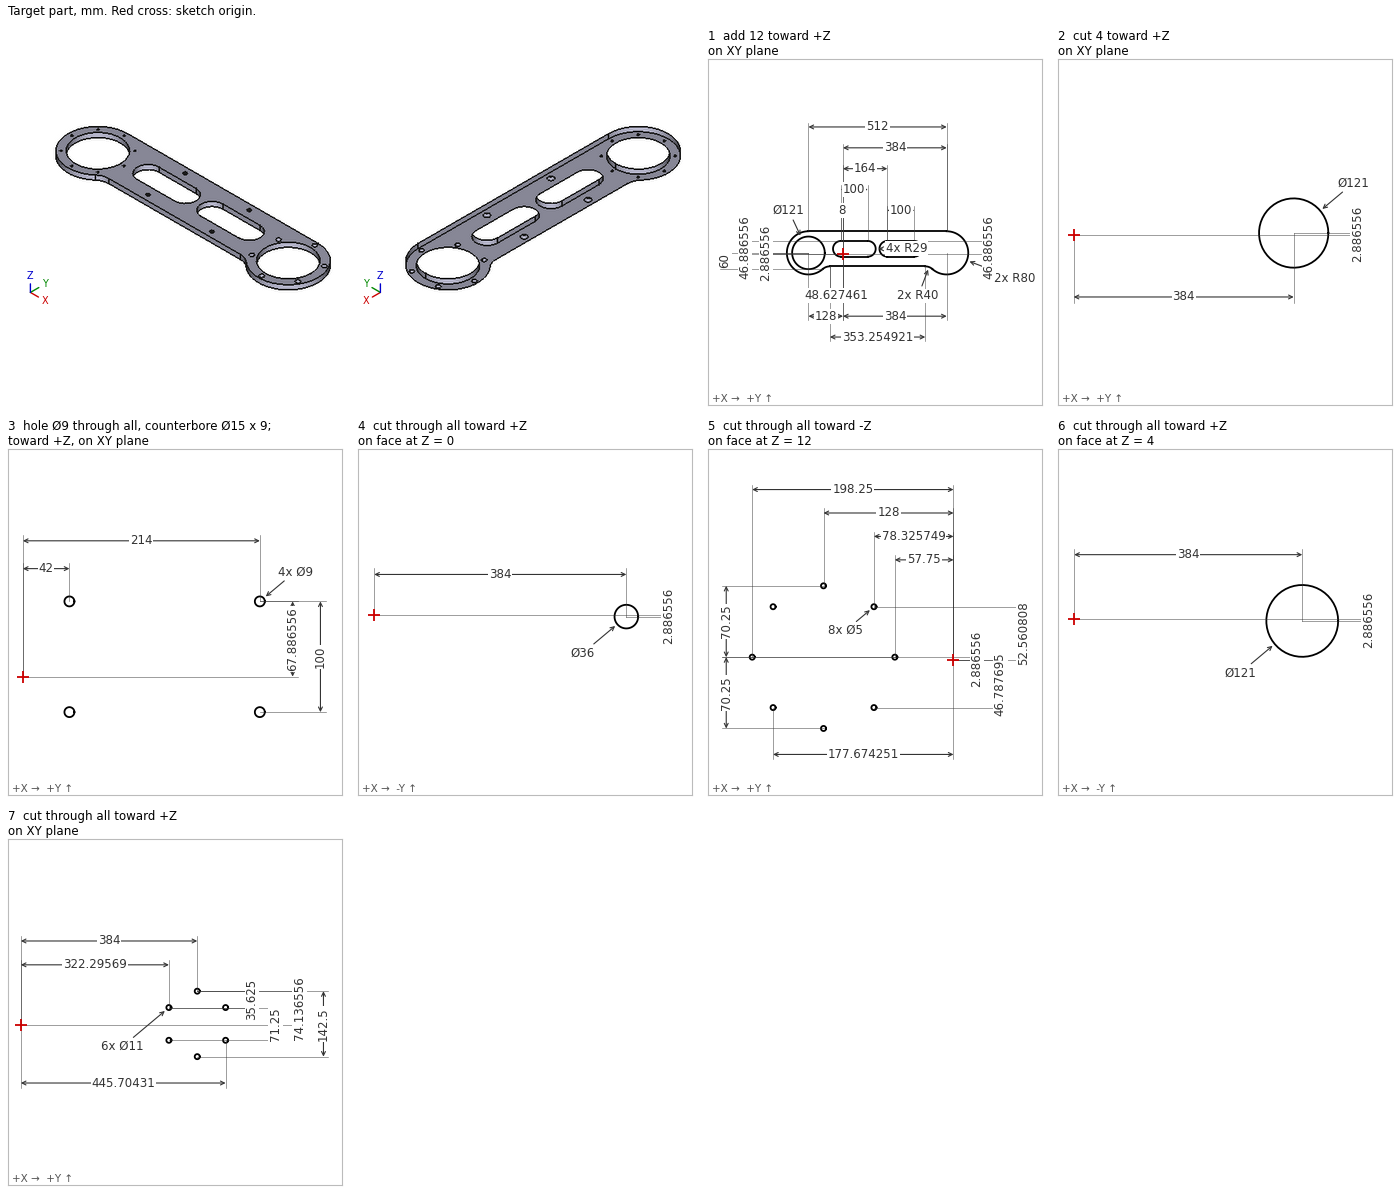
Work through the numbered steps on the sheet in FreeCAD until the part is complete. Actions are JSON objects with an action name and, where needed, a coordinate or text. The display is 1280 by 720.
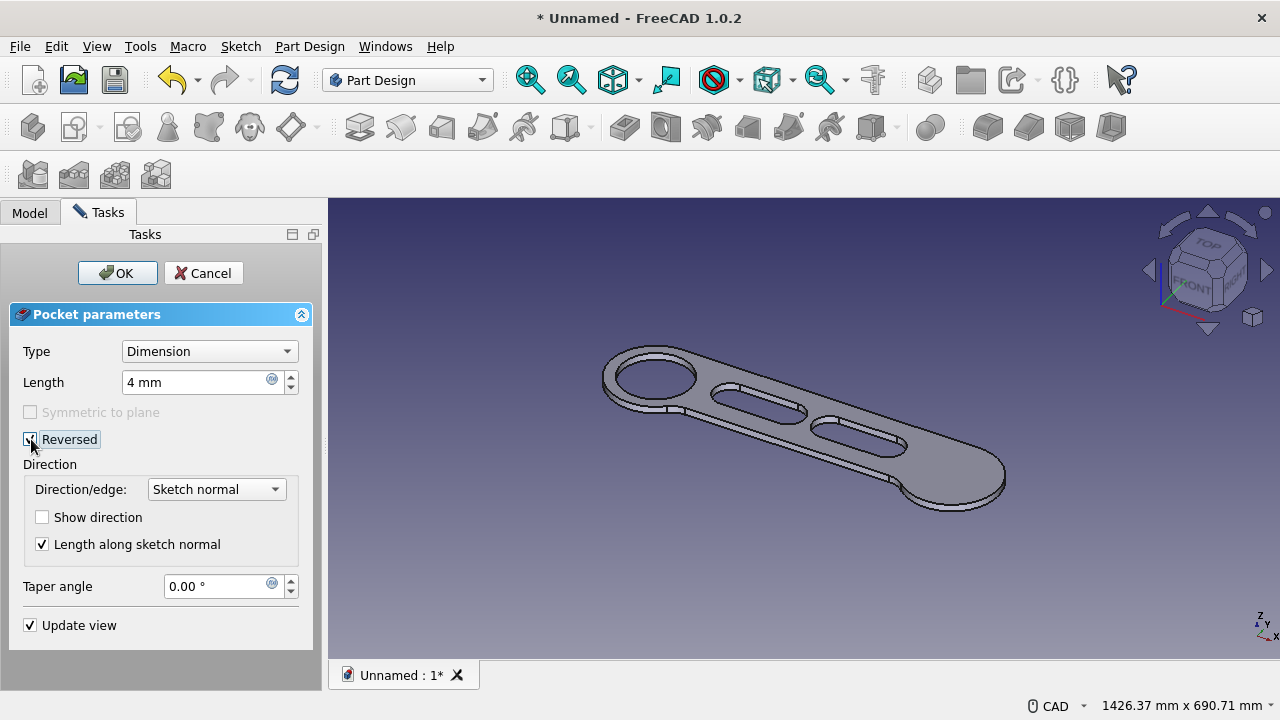
{"action": "left_click", "coordinate": [118, 273]}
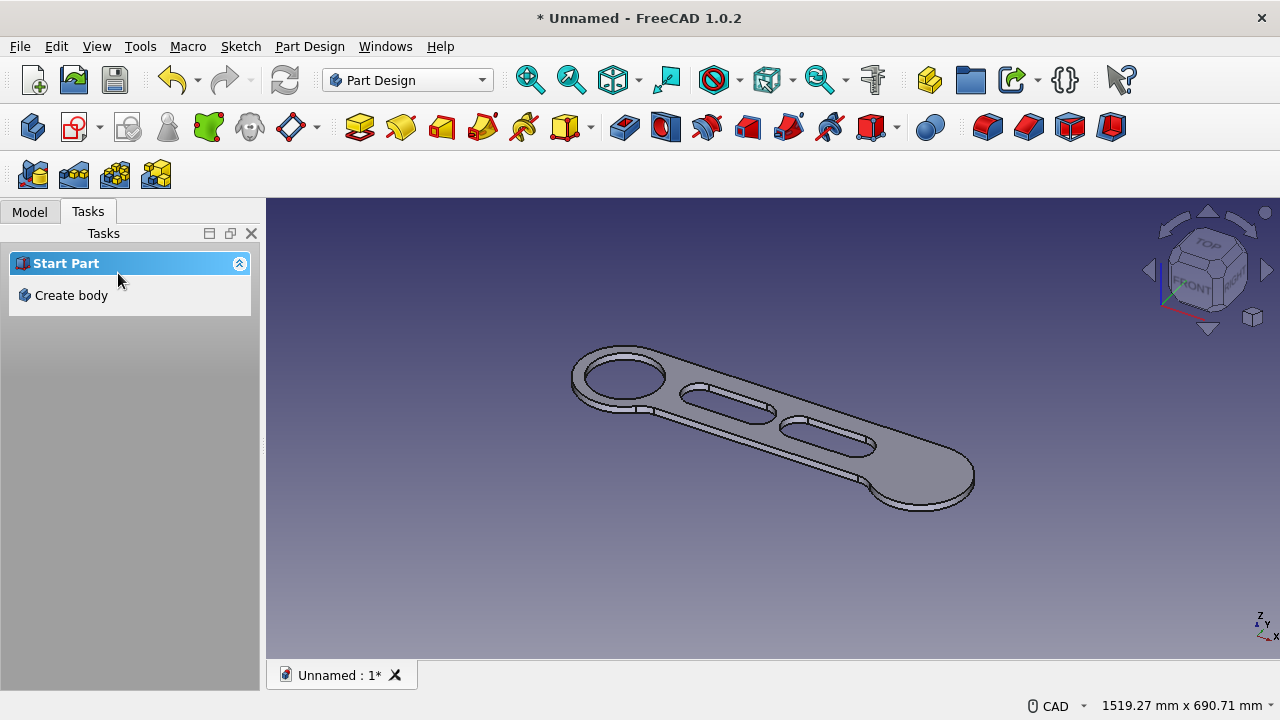
{"action": "left_click", "coordinate": [531, 80]}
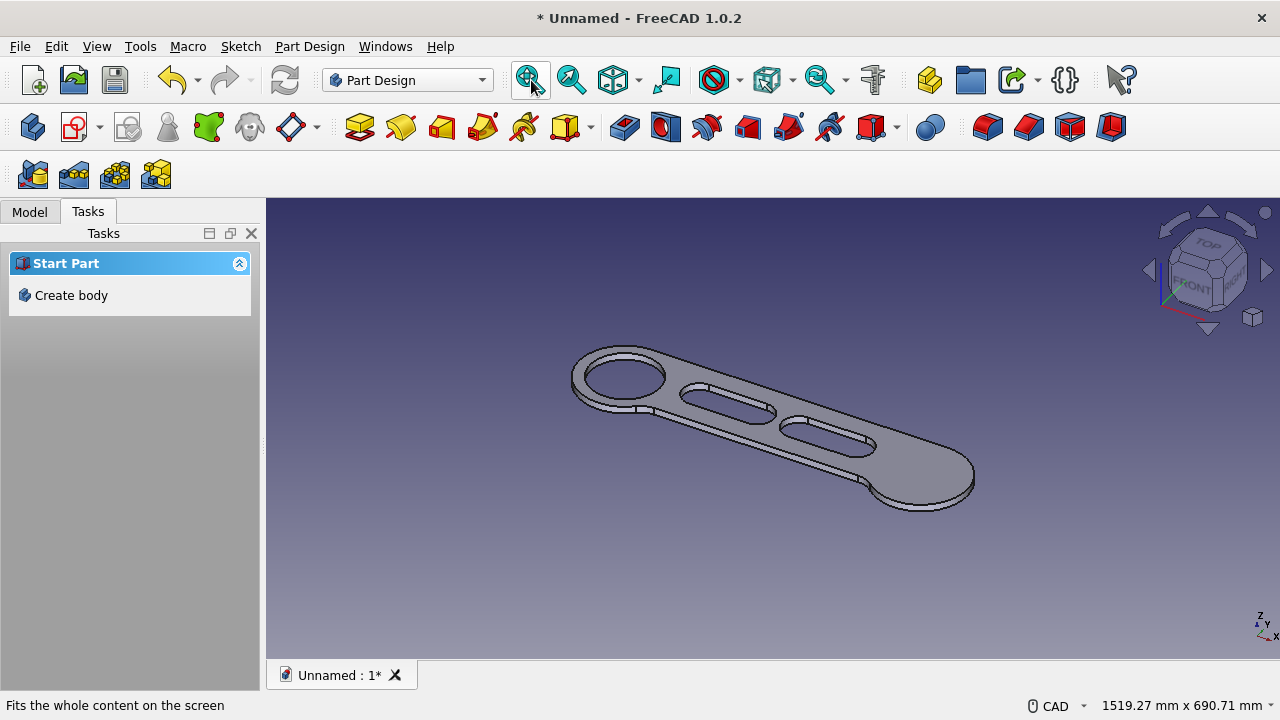
{"action": "left_click", "coordinate": [74, 128]}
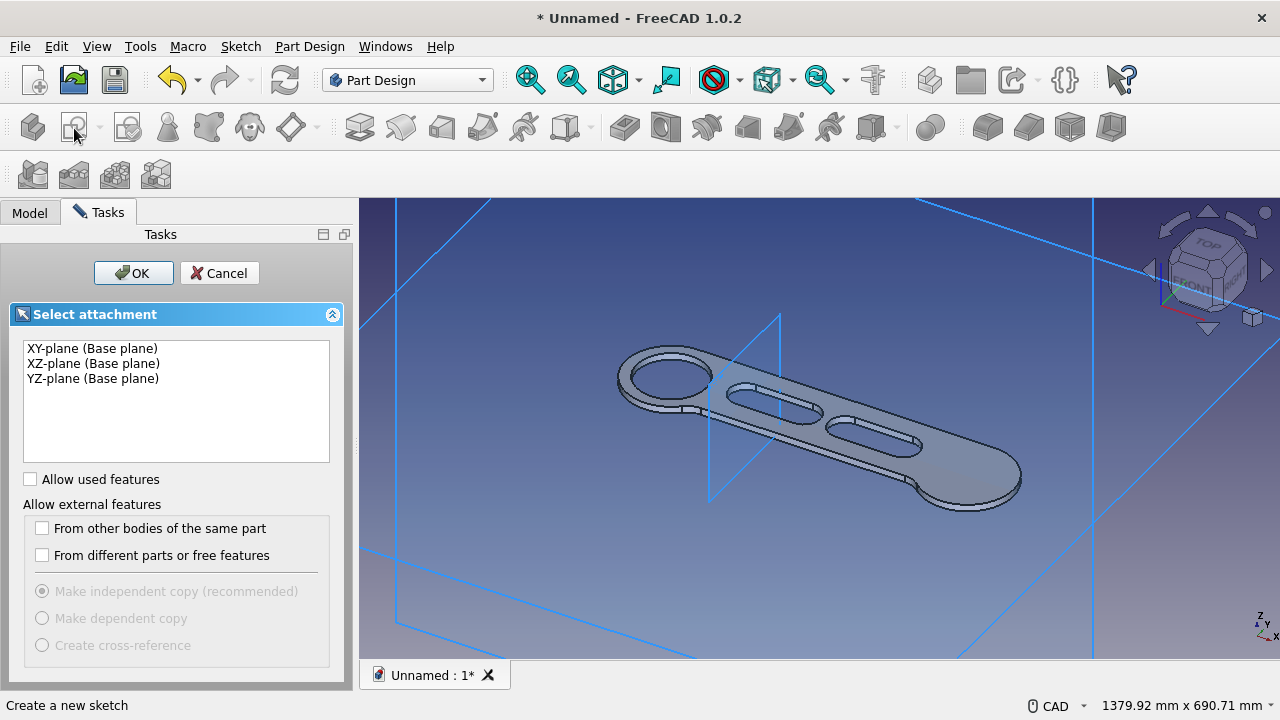
{"action": "left_click", "coordinate": [84, 348]}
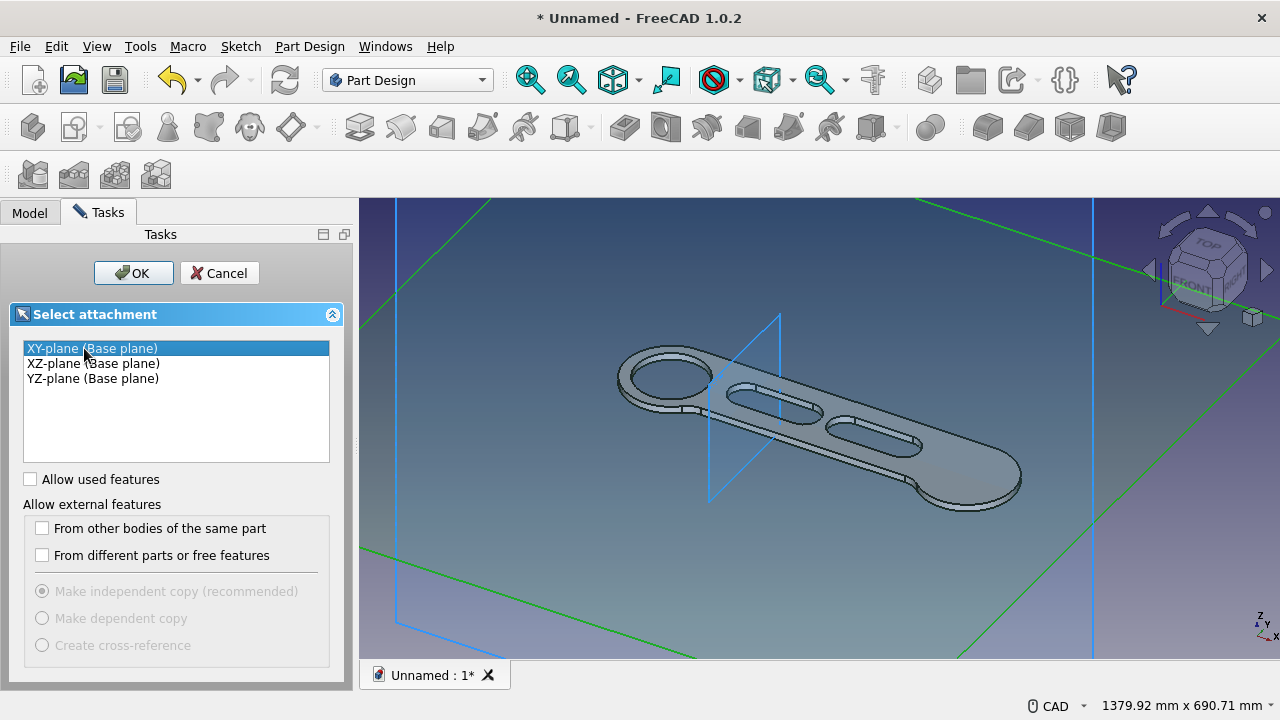
{"action": "left_click", "coordinate": [134, 273]}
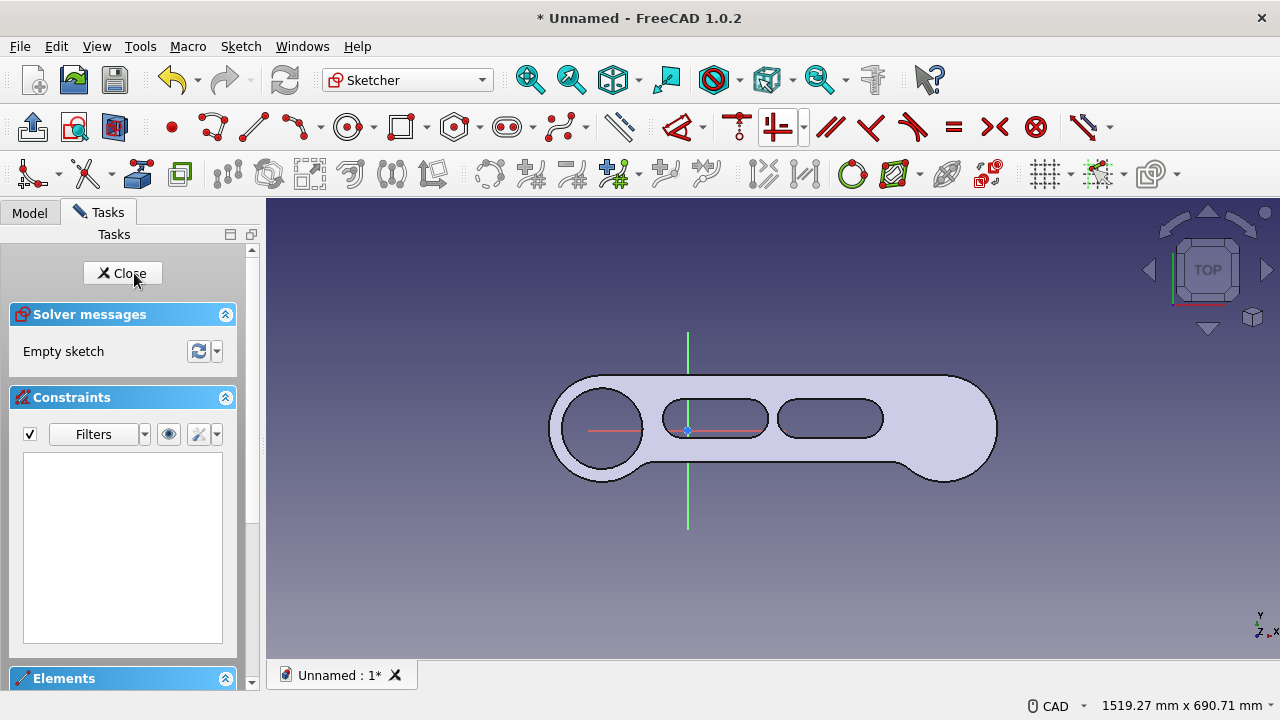
{"action": "left_click", "coordinate": [115, 128]}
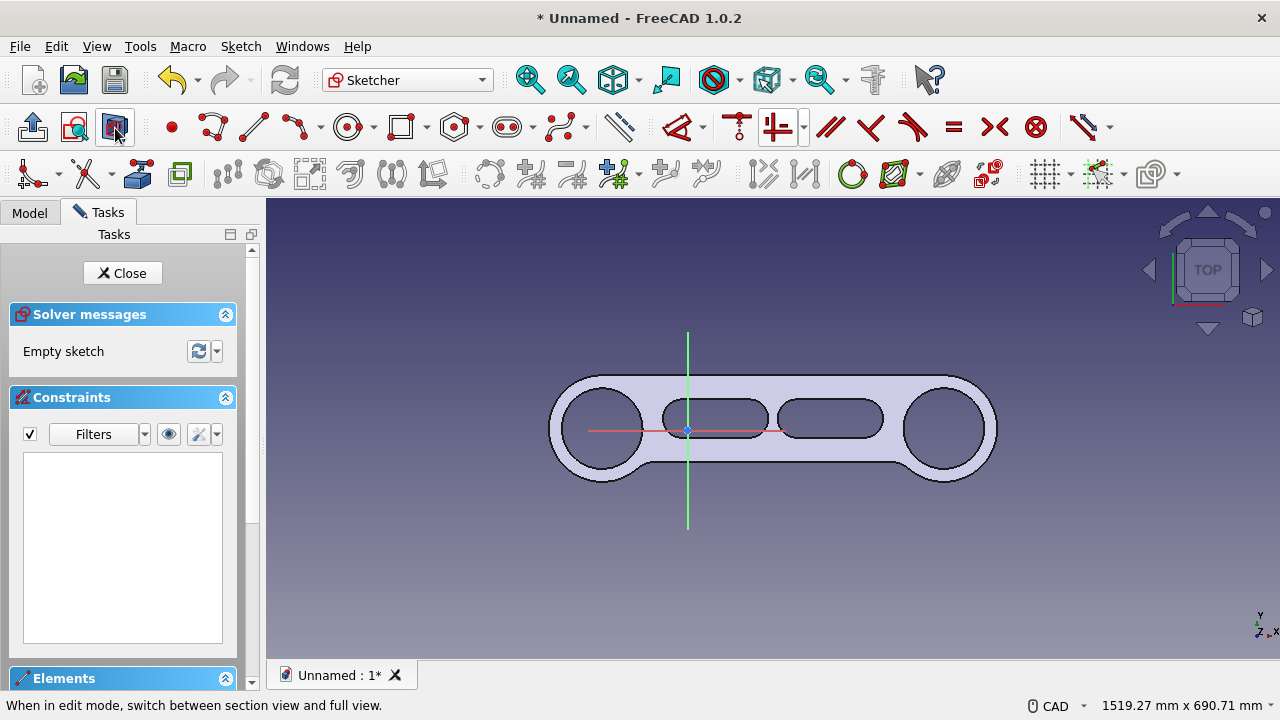
{"action": "scroll", "coordinate": [779, 415], "scroll_direction": "up", "scroll_amount": 7}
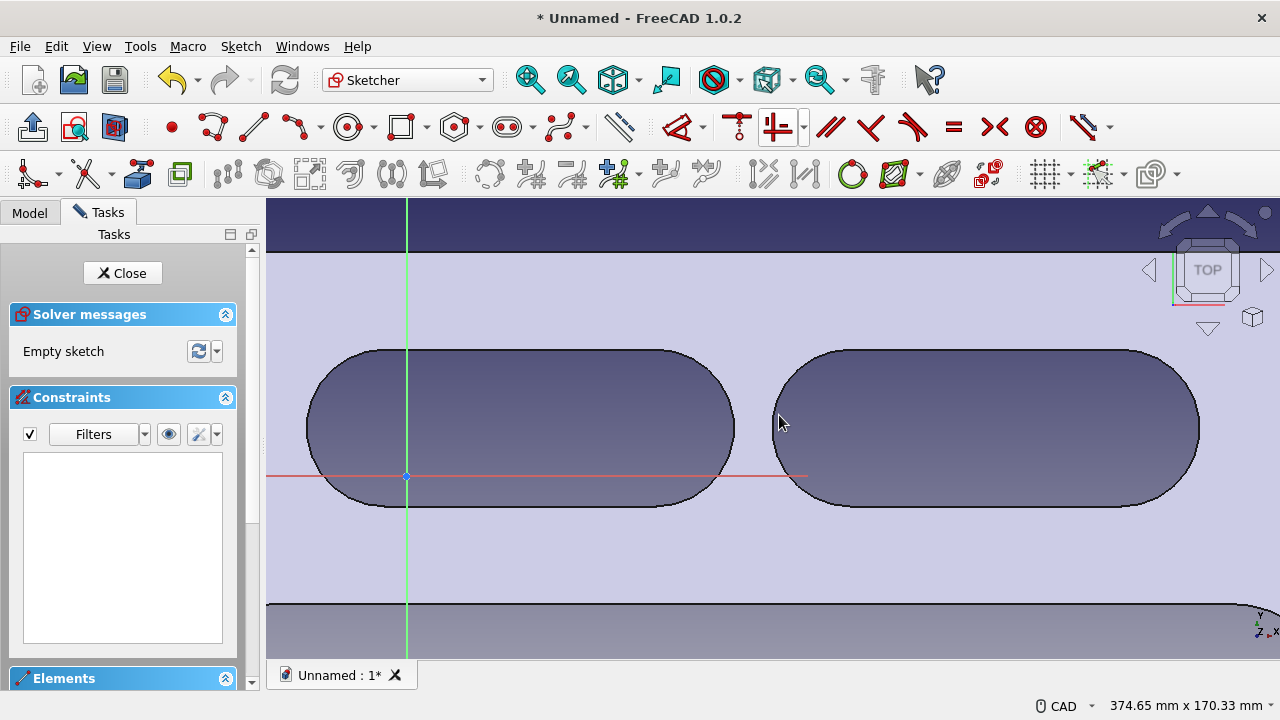
{"action": "left_click", "coordinate": [348, 128]}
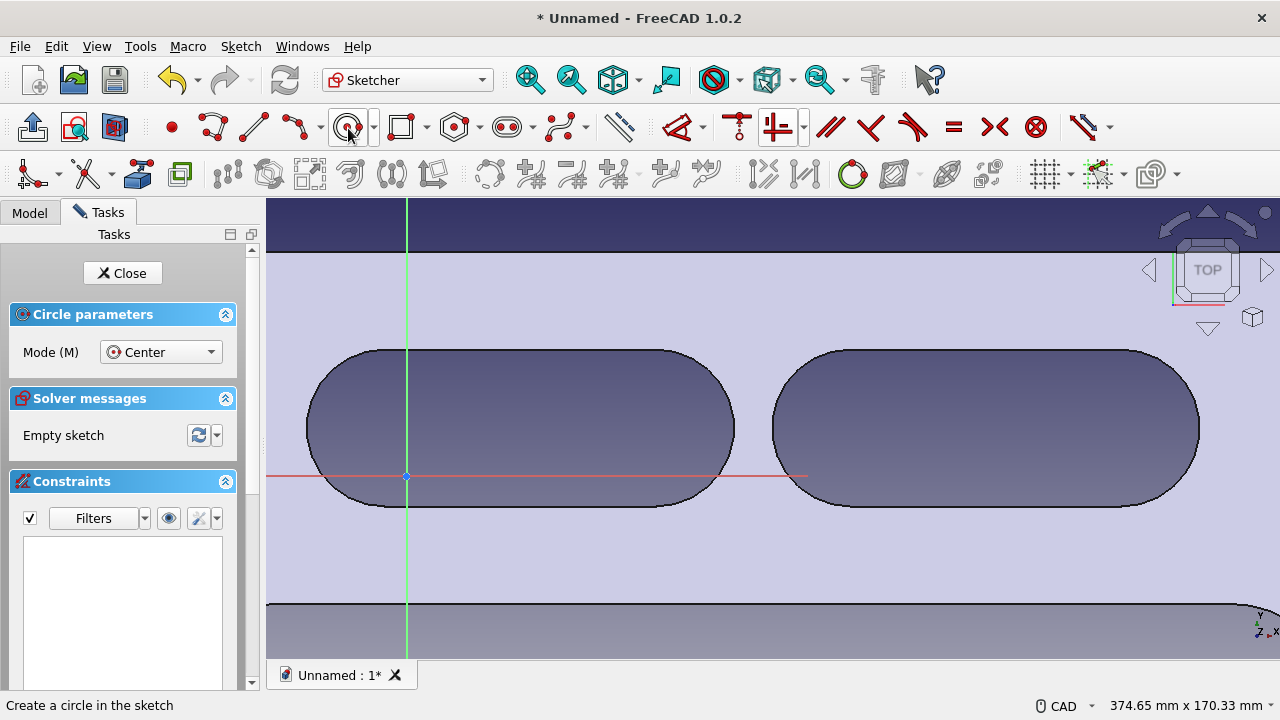
{"action": "scroll", "coordinate": [986, 293], "scroll_direction": "up", "scroll_amount": 4}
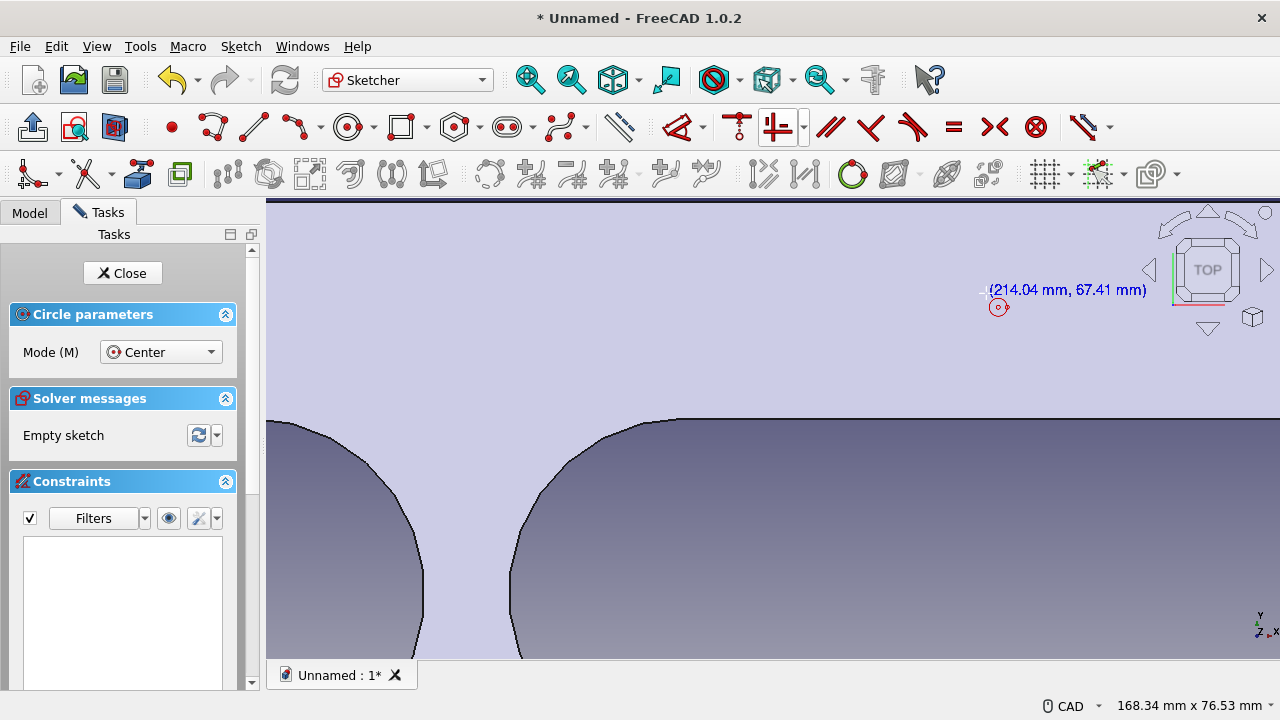
{"action": "left_click", "coordinate": [985, 292]}
{"action": "left_click", "coordinate": [1004, 273]}